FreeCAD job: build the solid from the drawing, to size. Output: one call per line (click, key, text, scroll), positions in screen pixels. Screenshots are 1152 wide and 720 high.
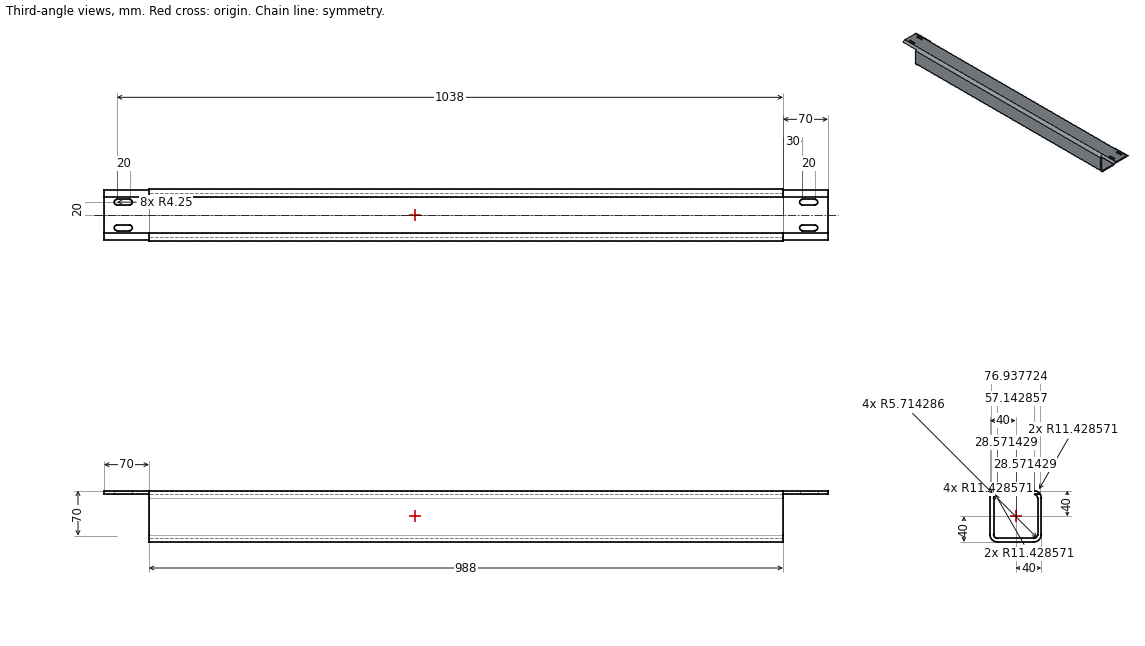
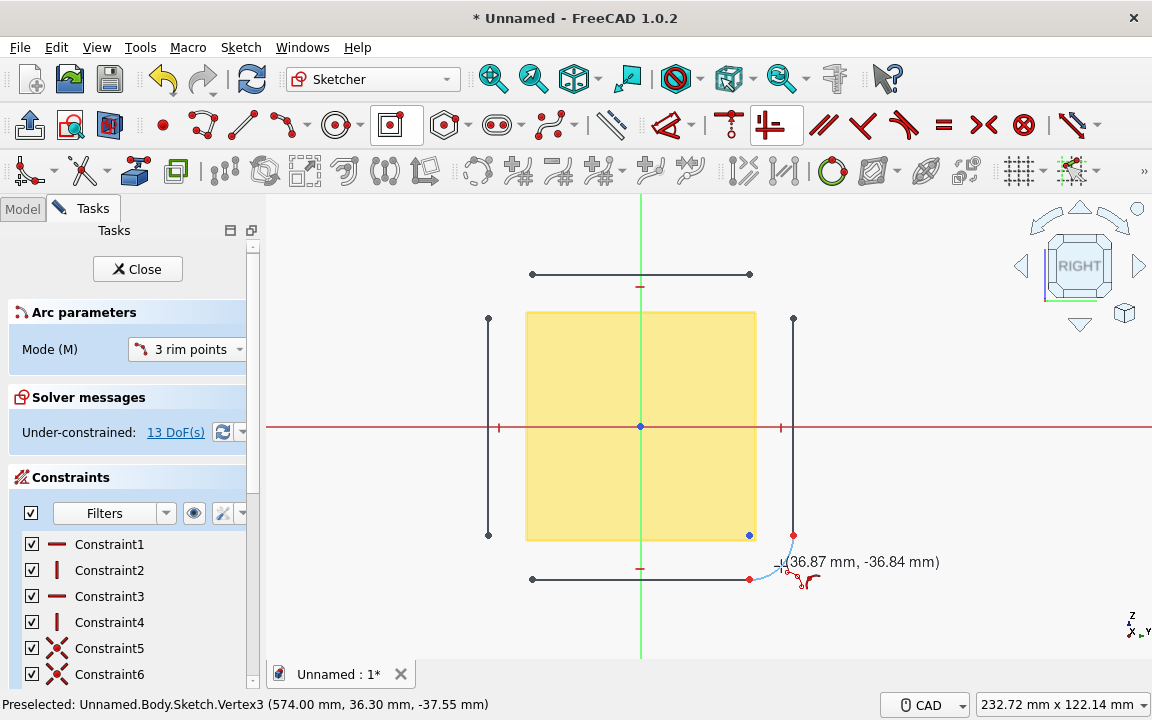
click(793, 319)
click(749, 275)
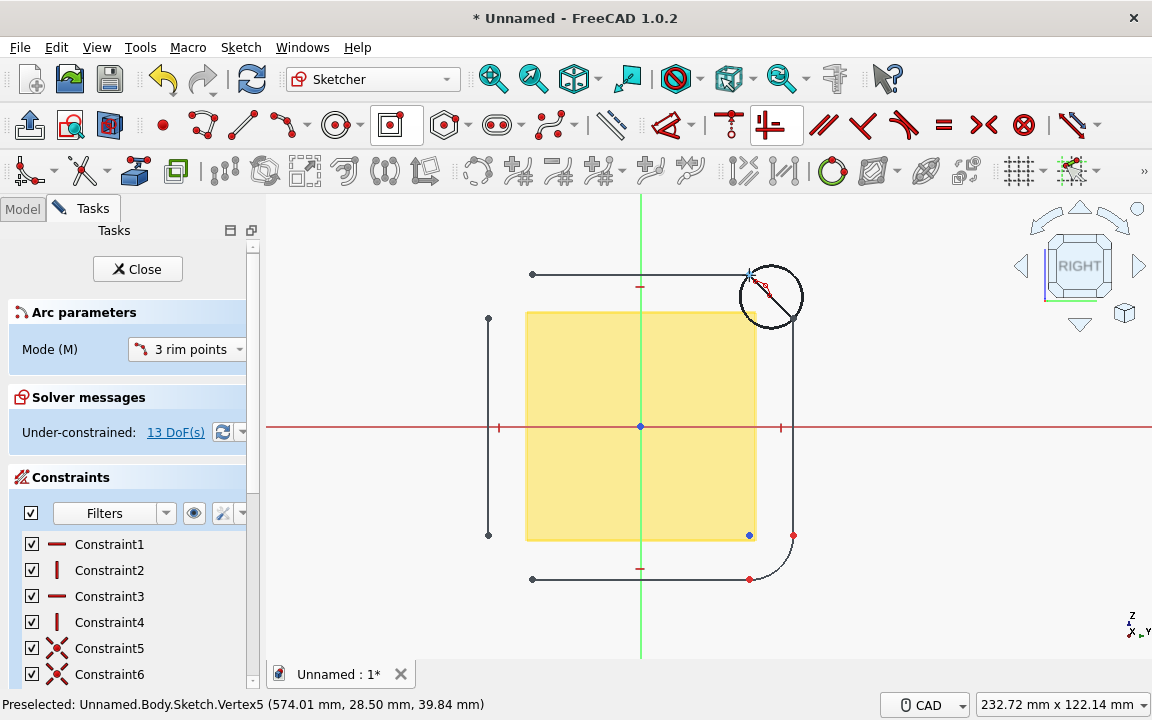
scroll(780, 287, up, 2)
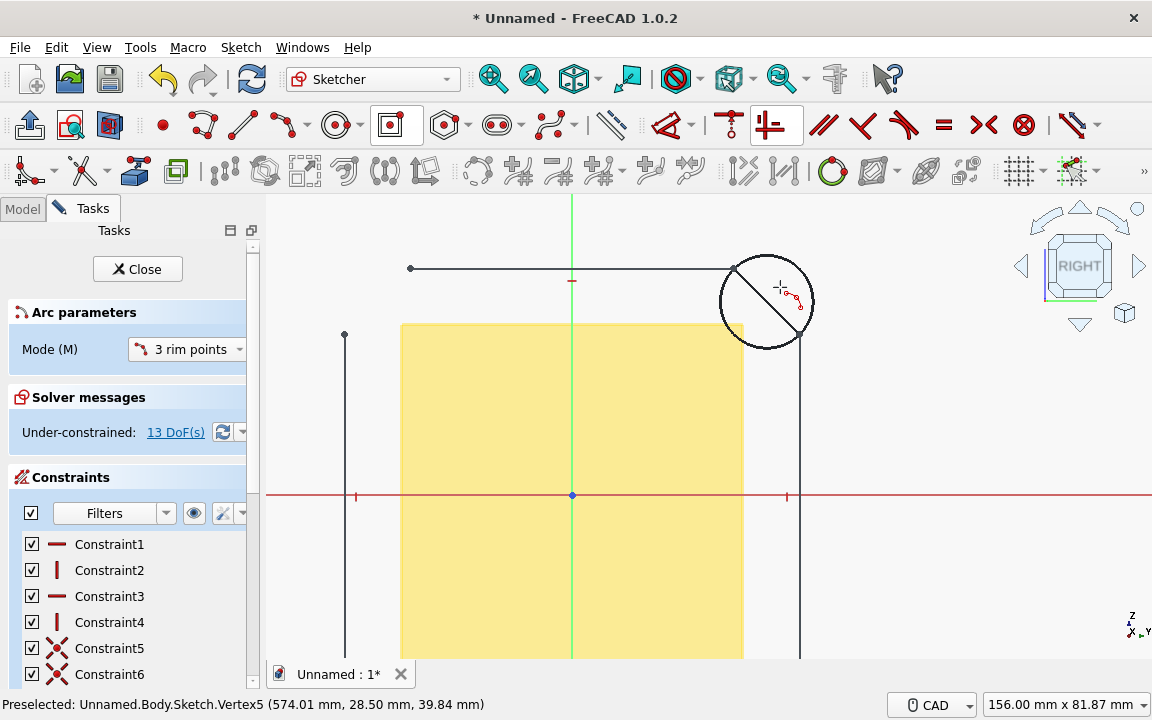
click(780, 287)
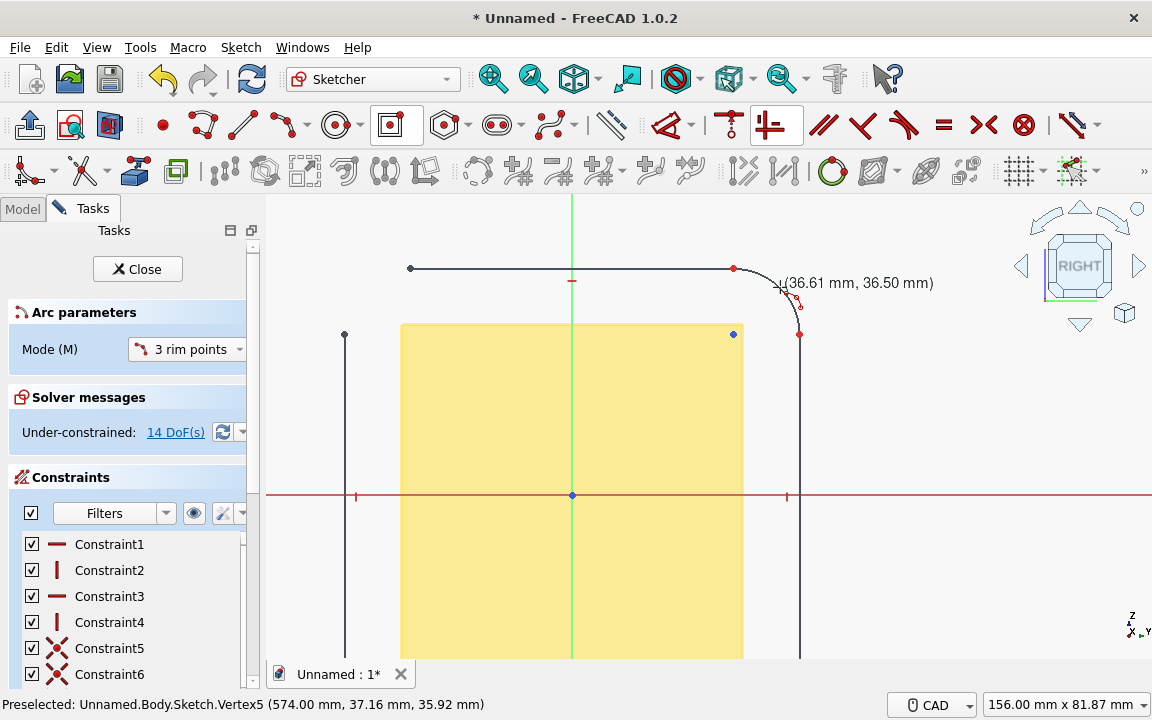
click(410, 269)
click(345, 335)
click(364, 287)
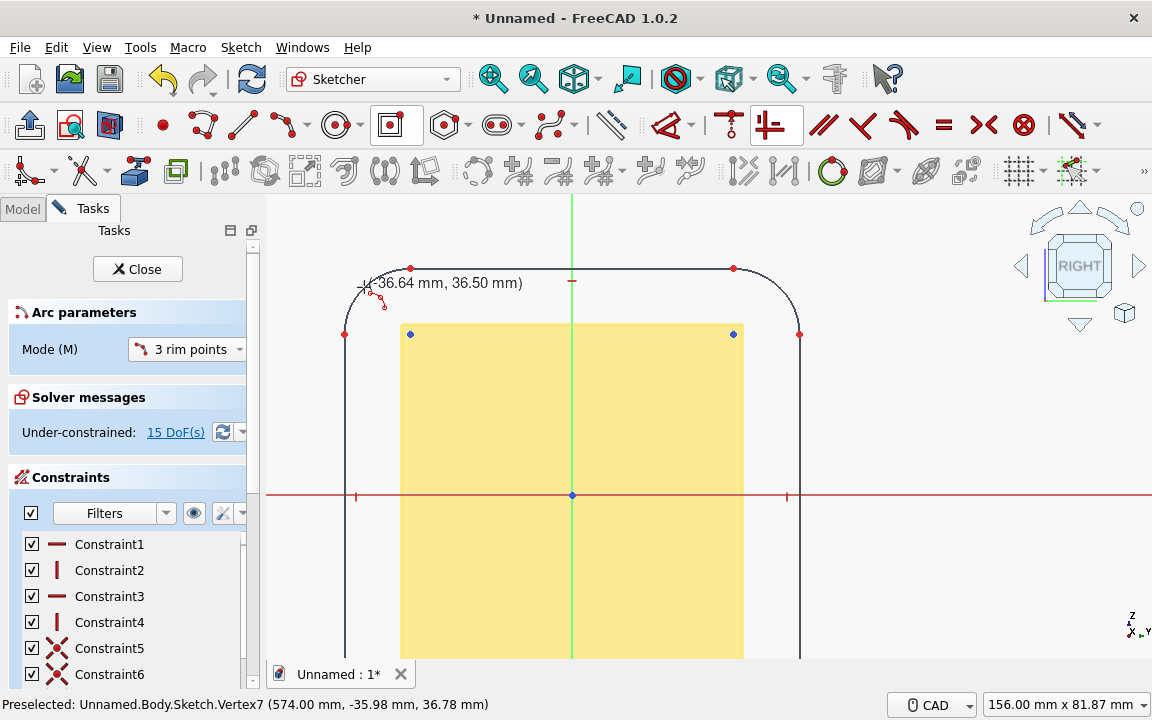
scroll(780, 287, down, 2)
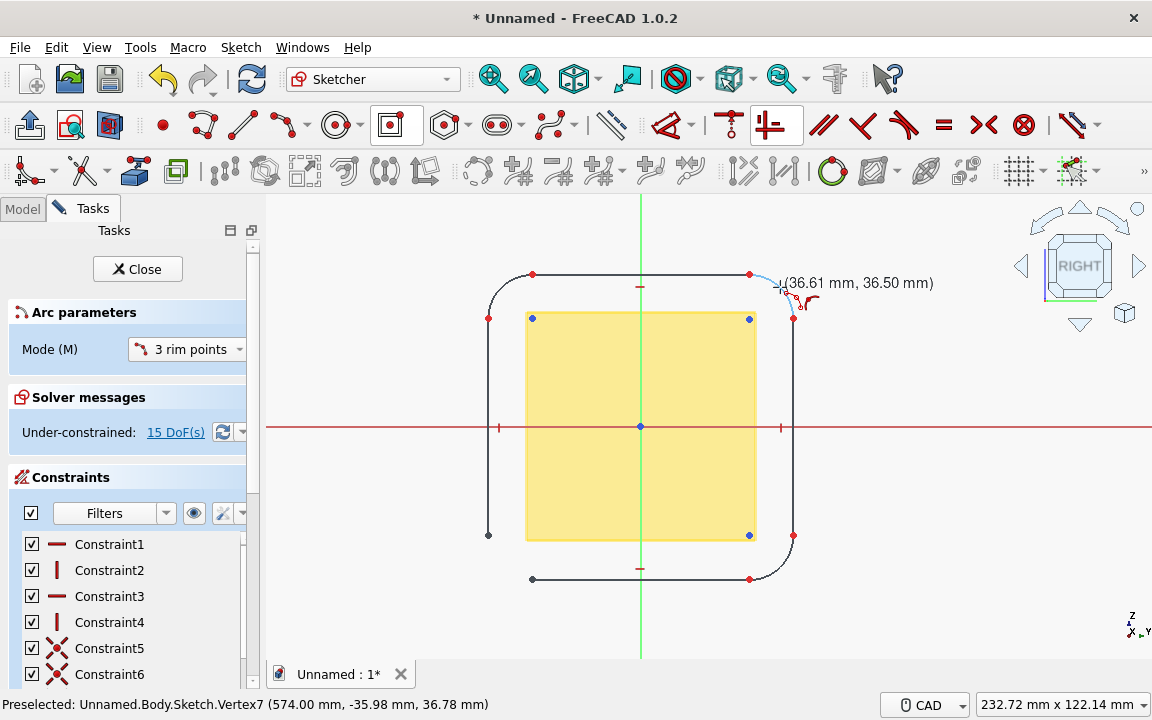
click(488, 536)
click(532, 580)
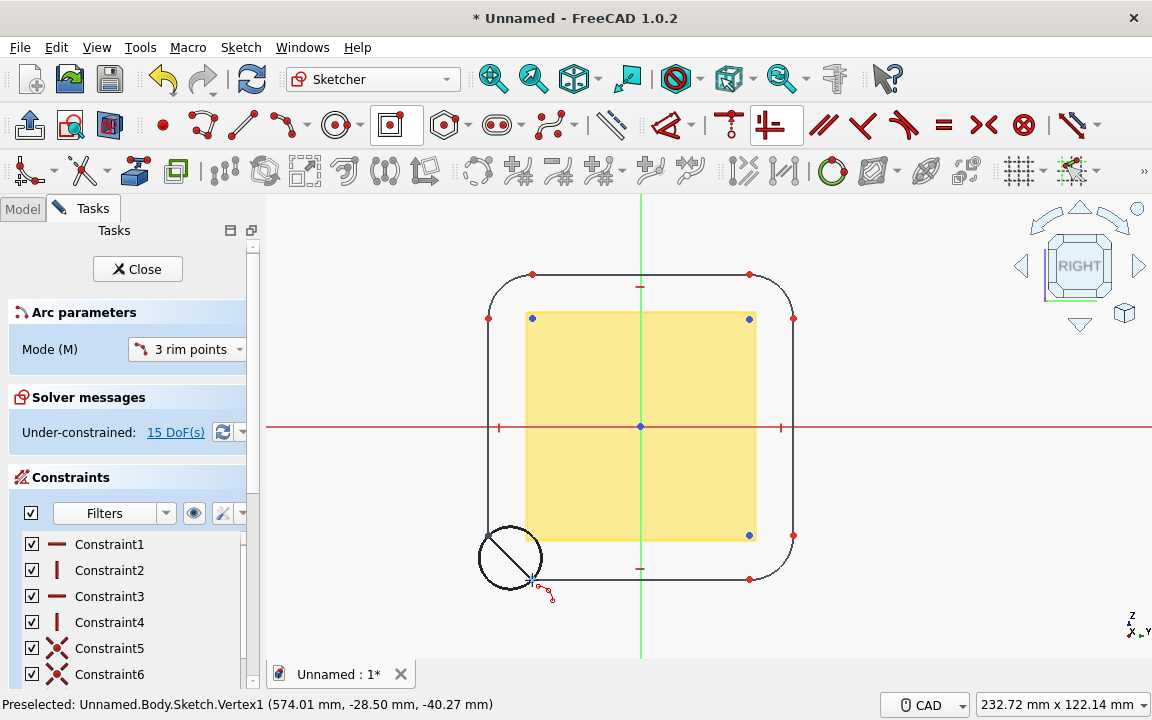
scroll(501, 566, up, 2)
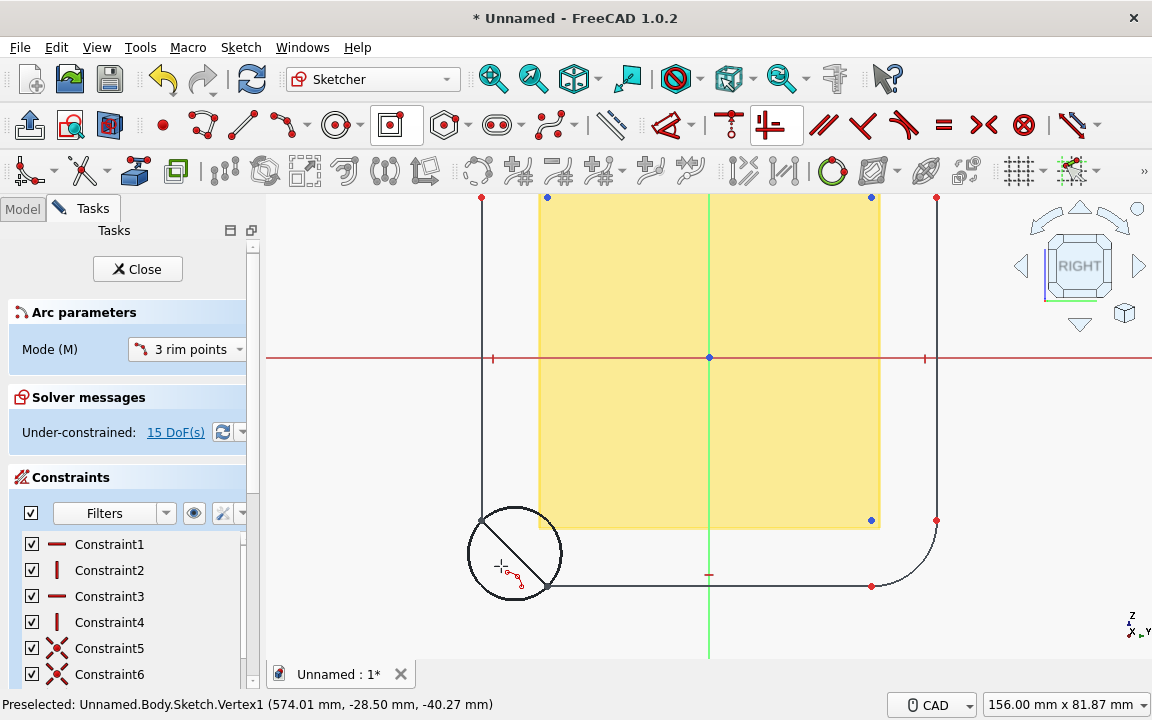
click(501, 566)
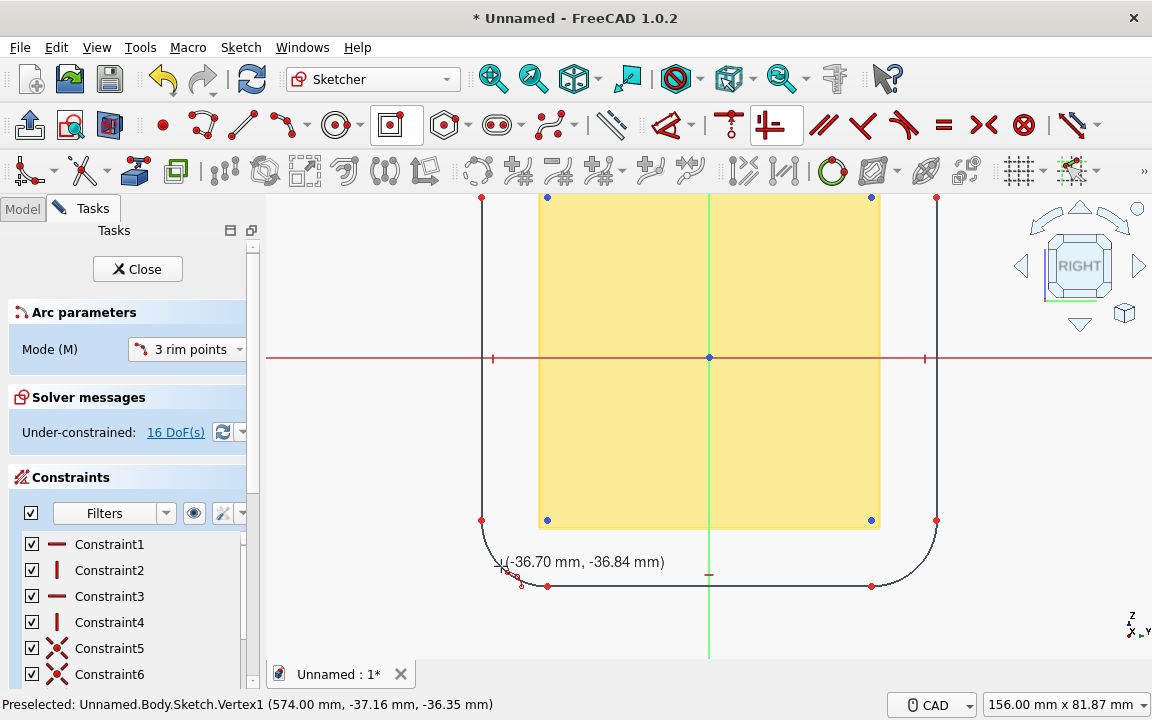
key(g)
key(l)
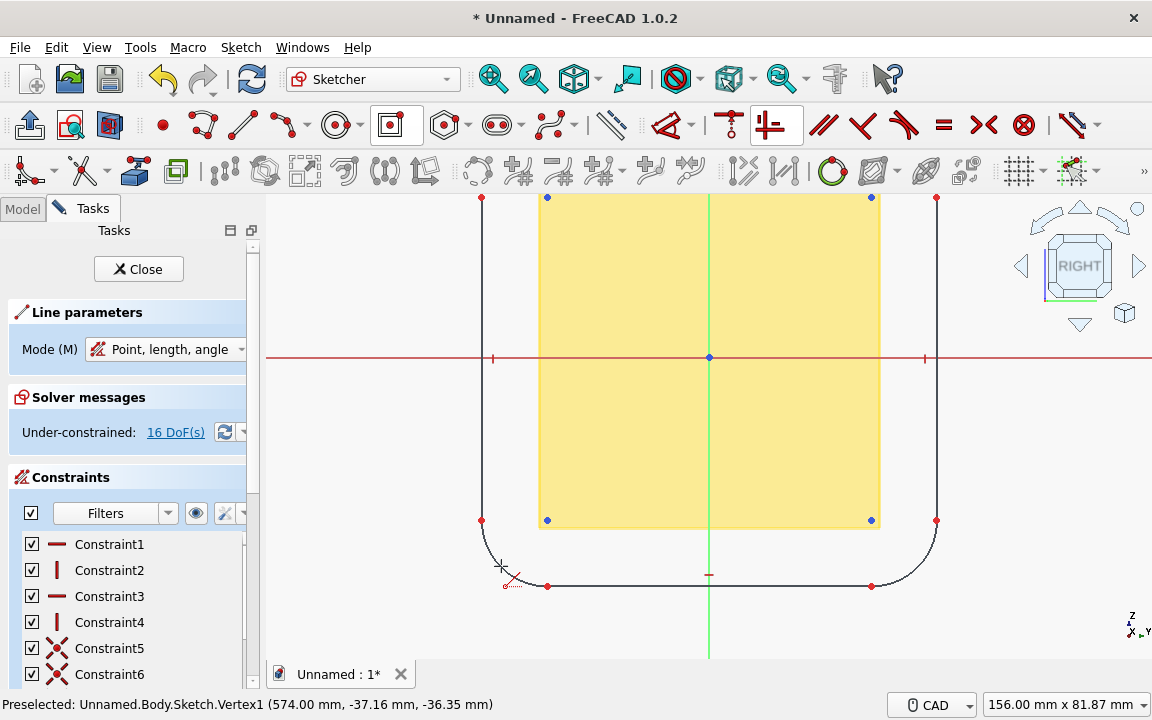
scroll(500, 566, down, 2)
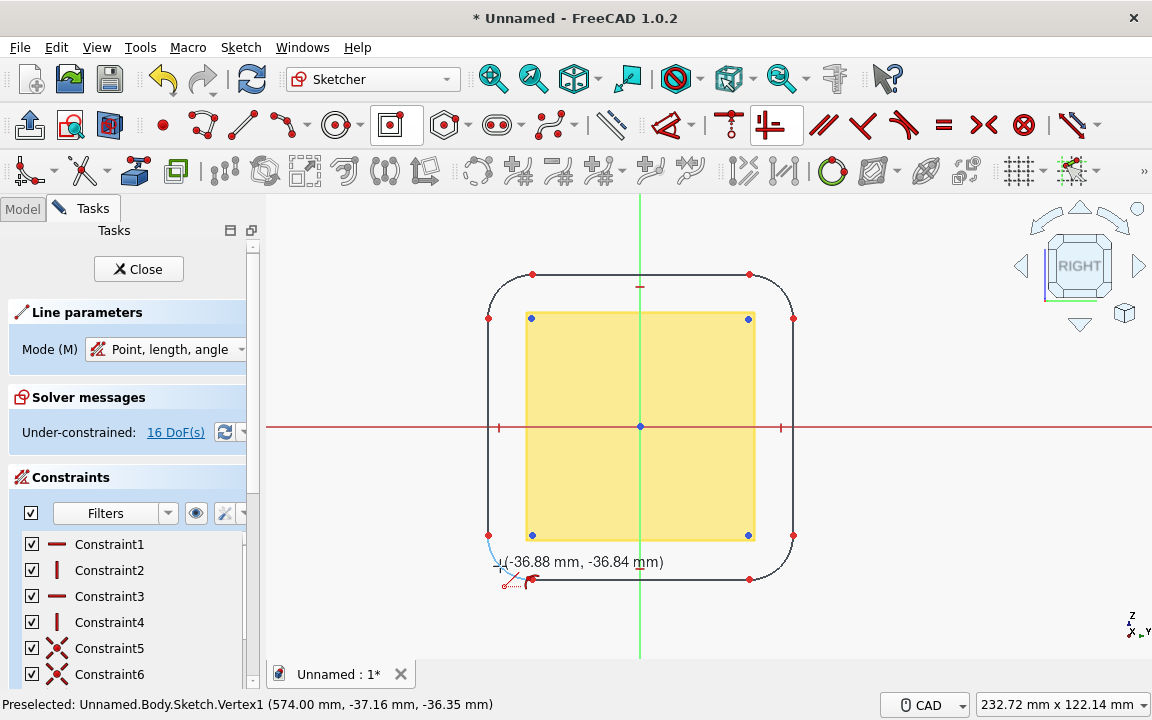
click(532, 296)
click(749, 296)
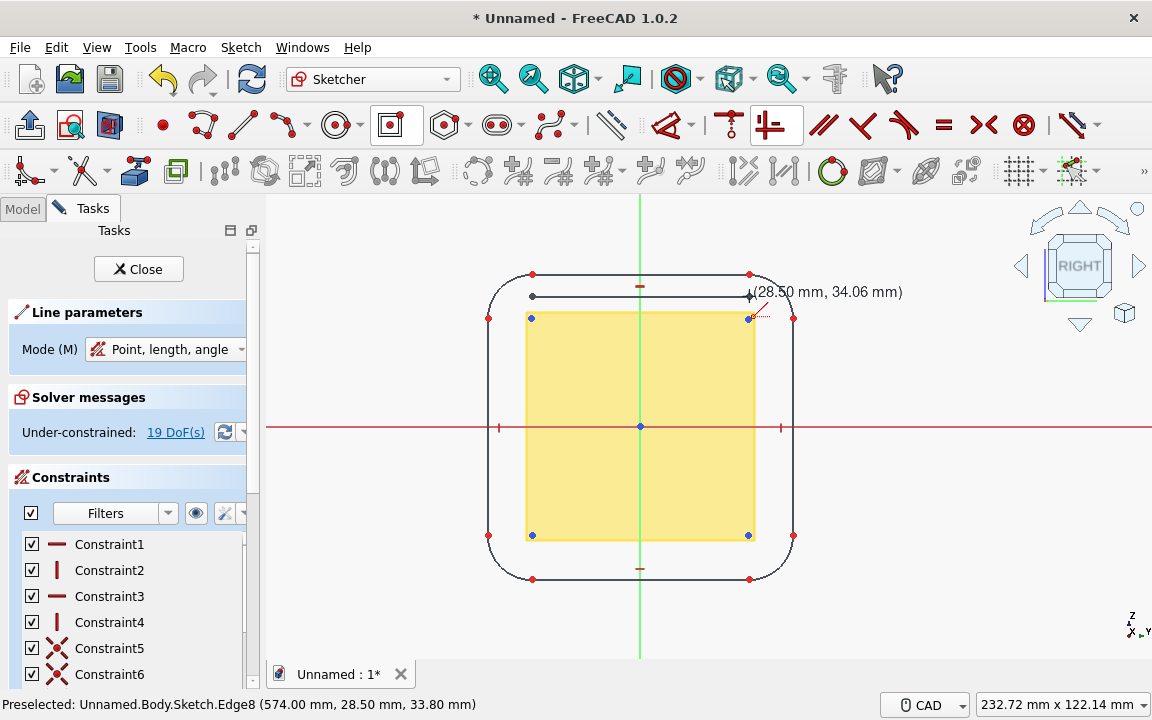
click(771, 318)
click(771, 535)